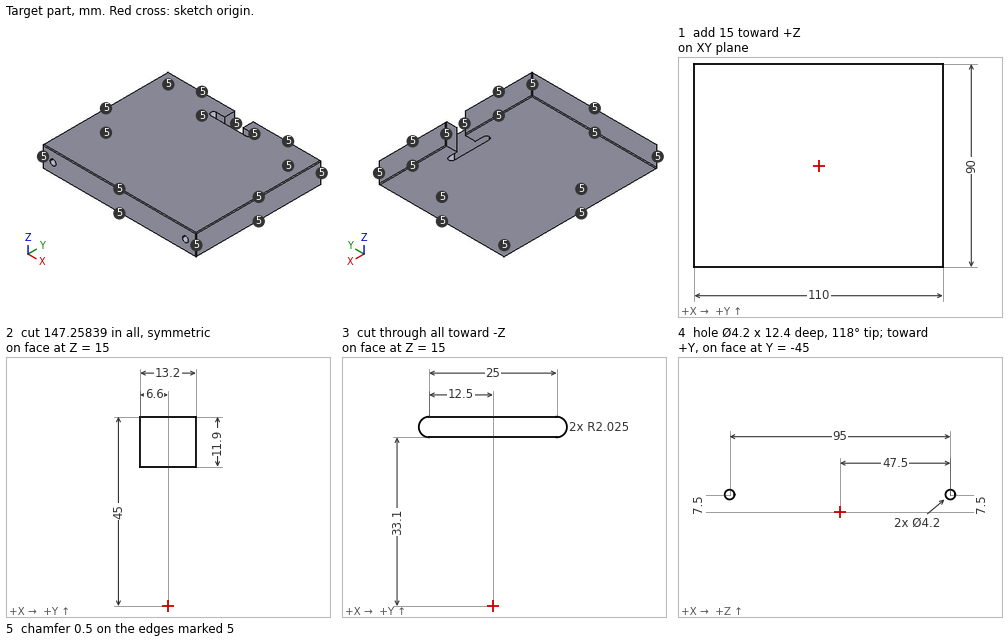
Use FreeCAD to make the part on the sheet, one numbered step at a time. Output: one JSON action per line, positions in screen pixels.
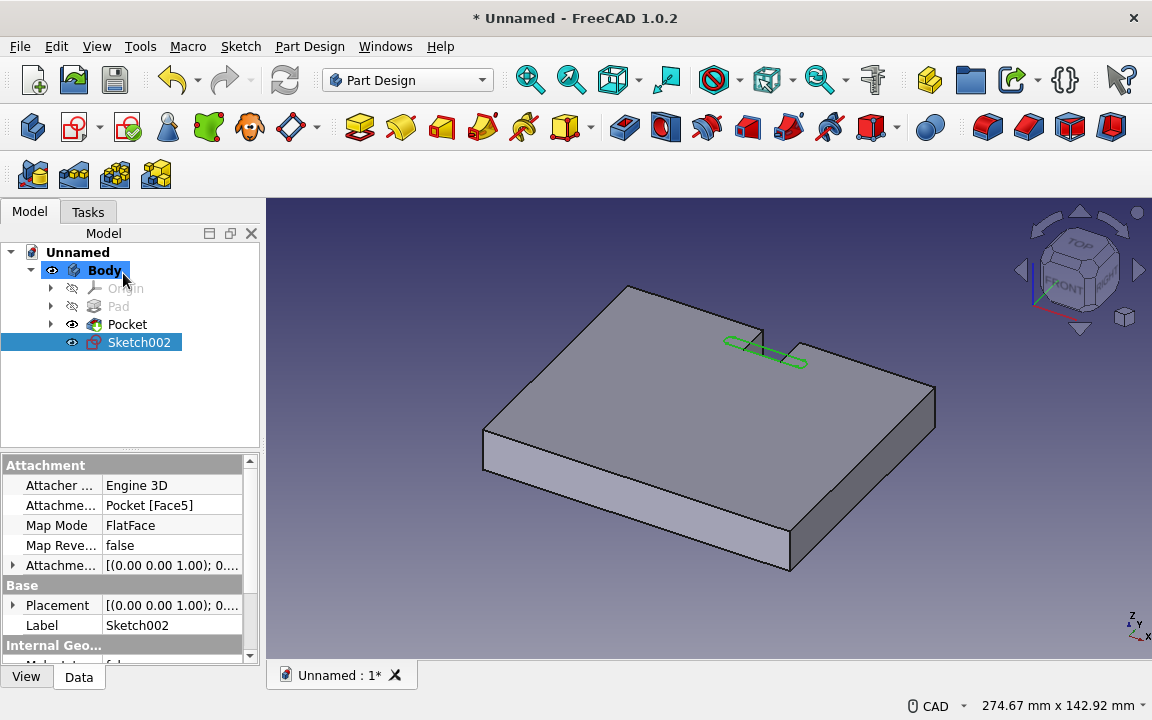
{"action": "left_click", "coordinate": [625, 128]}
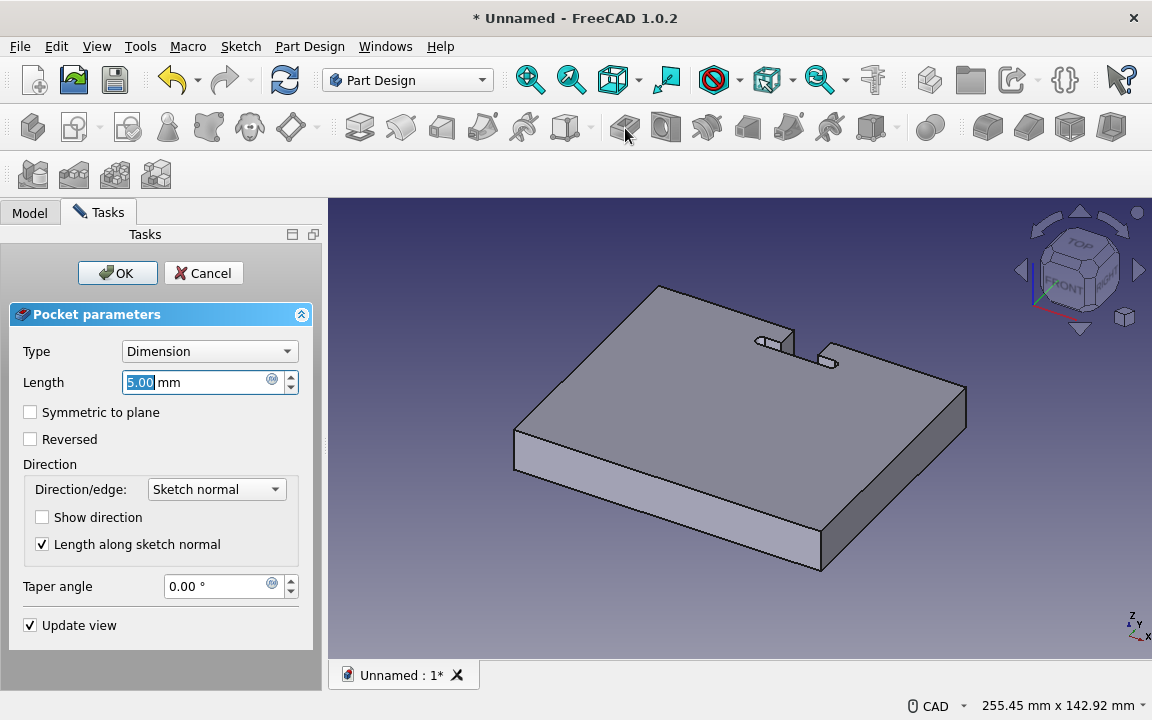
{"action": "left_click", "coordinate": [210, 352]}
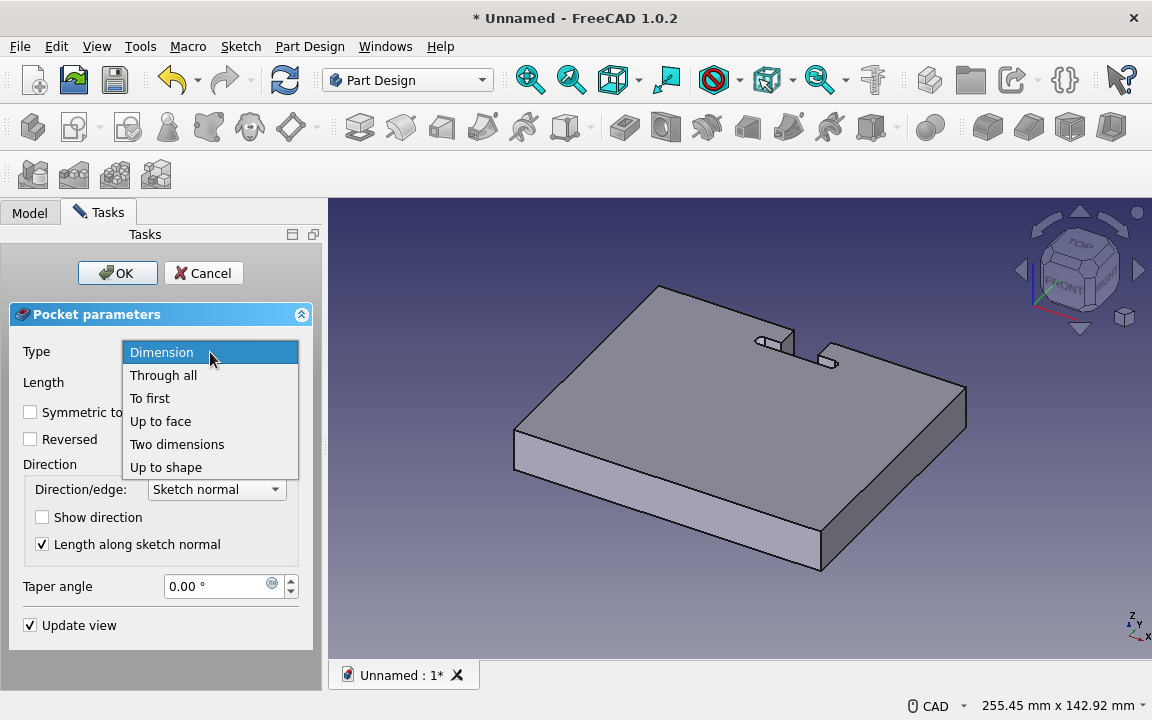
{"action": "left_click", "coordinate": [208, 376]}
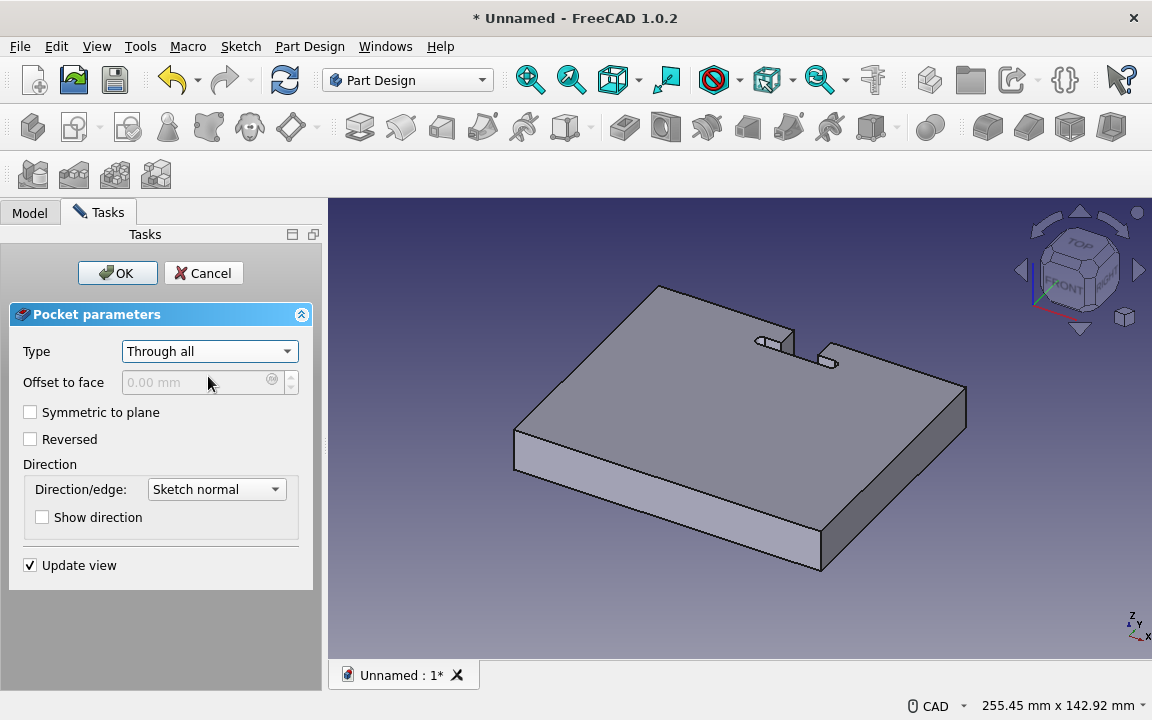
{"action": "left_click", "coordinate": [118, 273]}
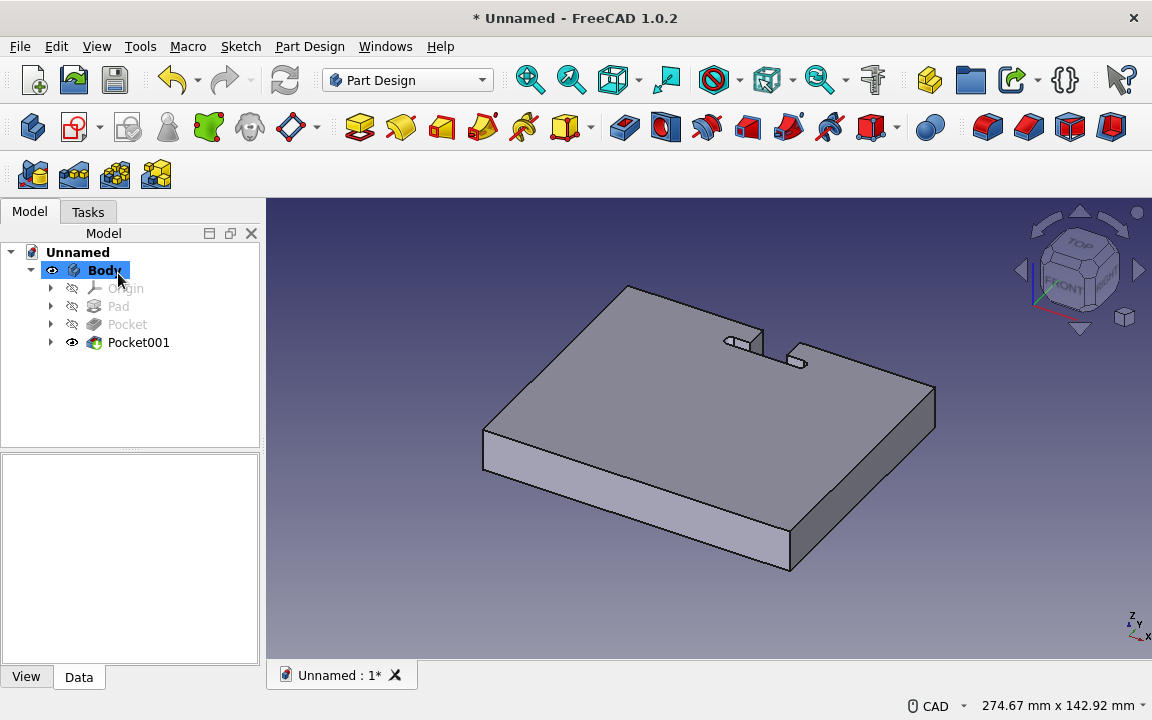
{"action": "left_click", "coordinate": [768, 543]}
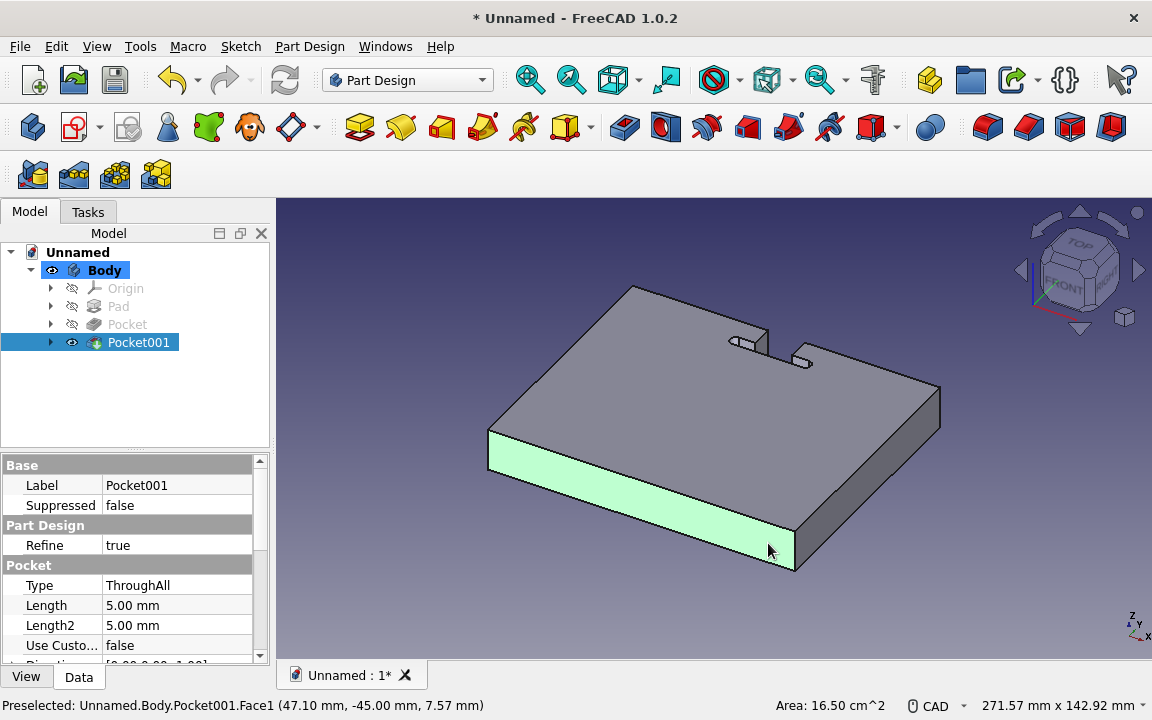
{"action": "left_click", "coordinate": [74, 128]}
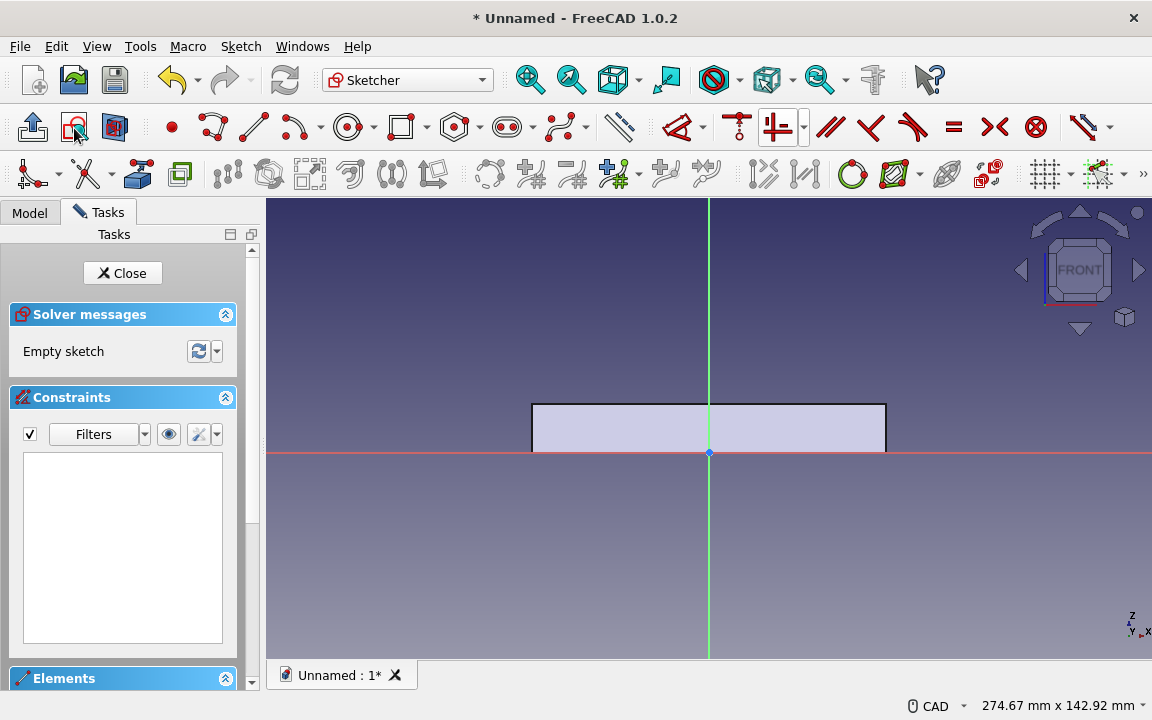
{"action": "scroll", "coordinate": [848, 455], "scroll_direction": "up", "scroll_amount": 2}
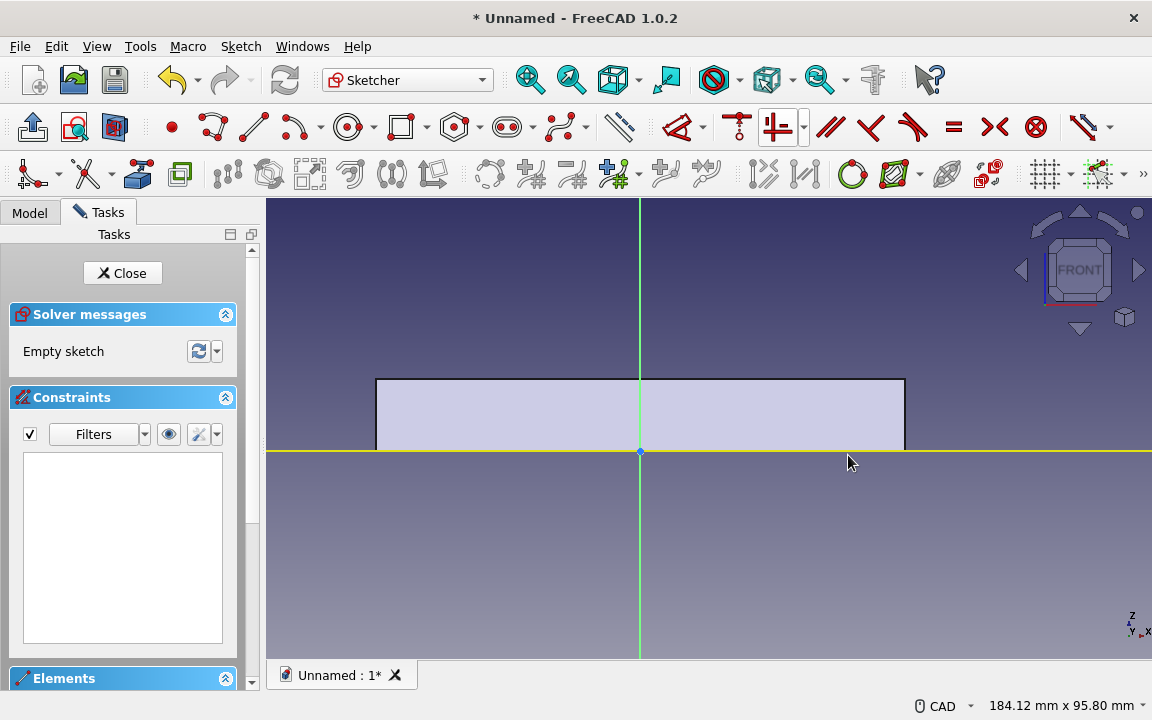
{"action": "left_click", "coordinate": [348, 128]}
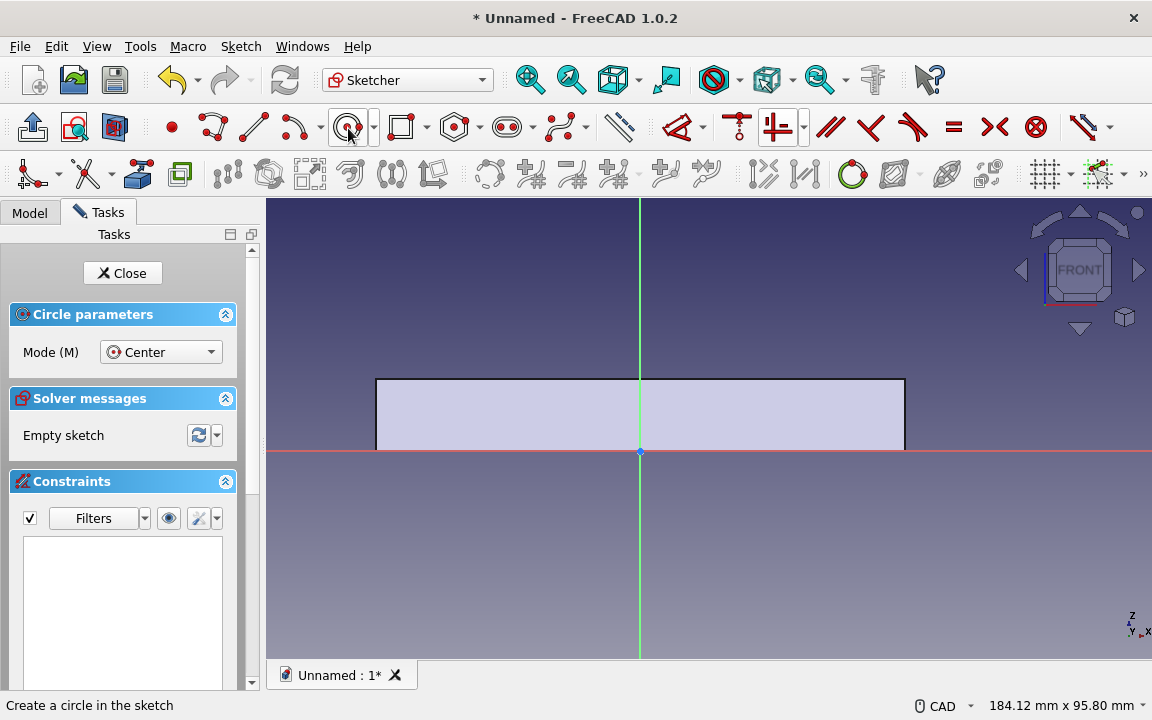
{"action": "scroll", "coordinate": [869, 415], "scroll_direction": "up", "scroll_amount": 5}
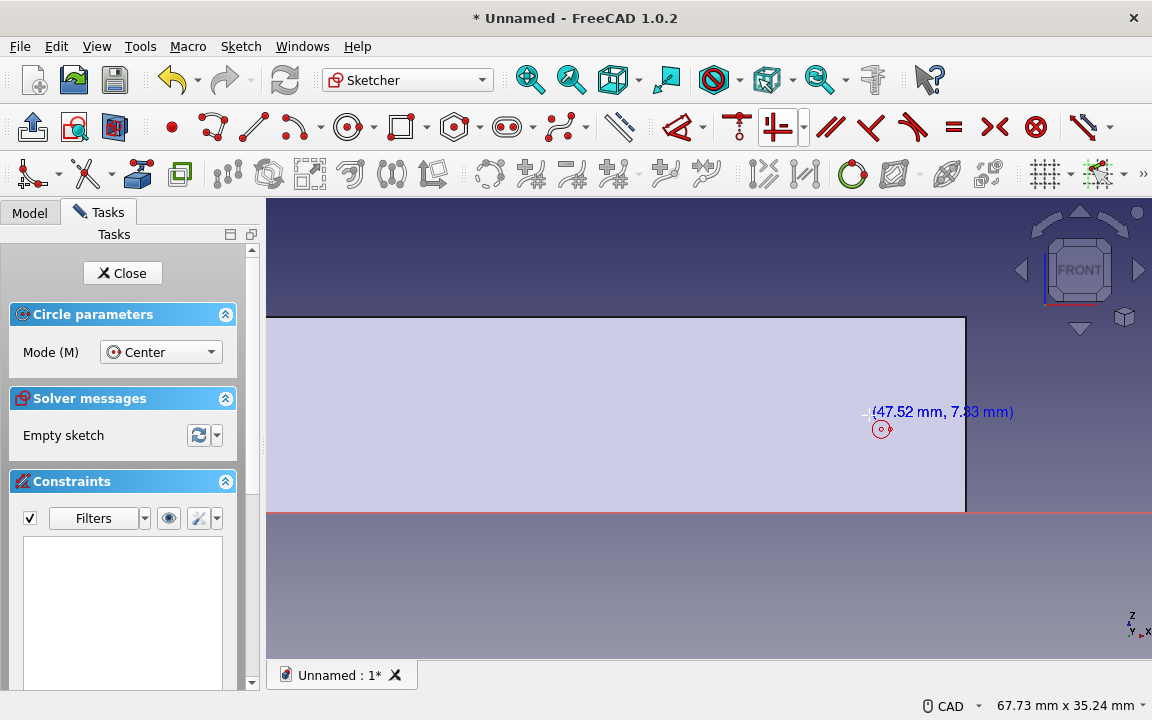
{"action": "left_click", "coordinate": [868, 415]}
{"action": "mouse_move", "coordinate": [887, 395]}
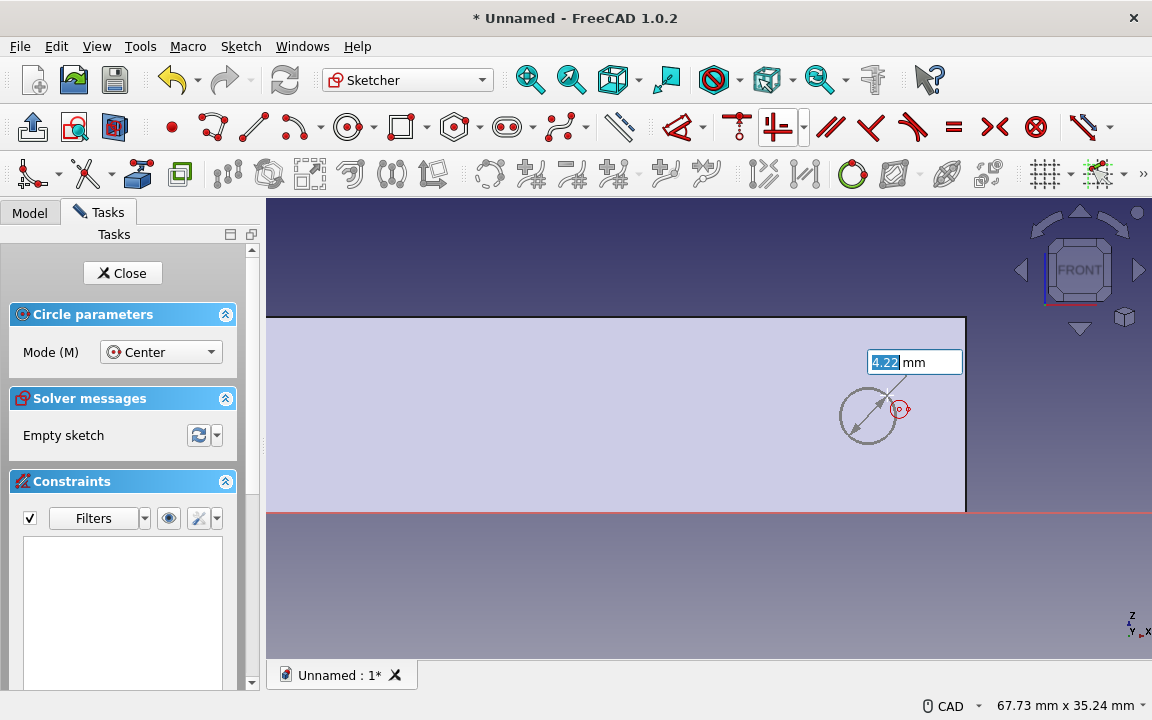
{"action": "type", "text": "4.2"}
{"action": "key", "text": "Return"}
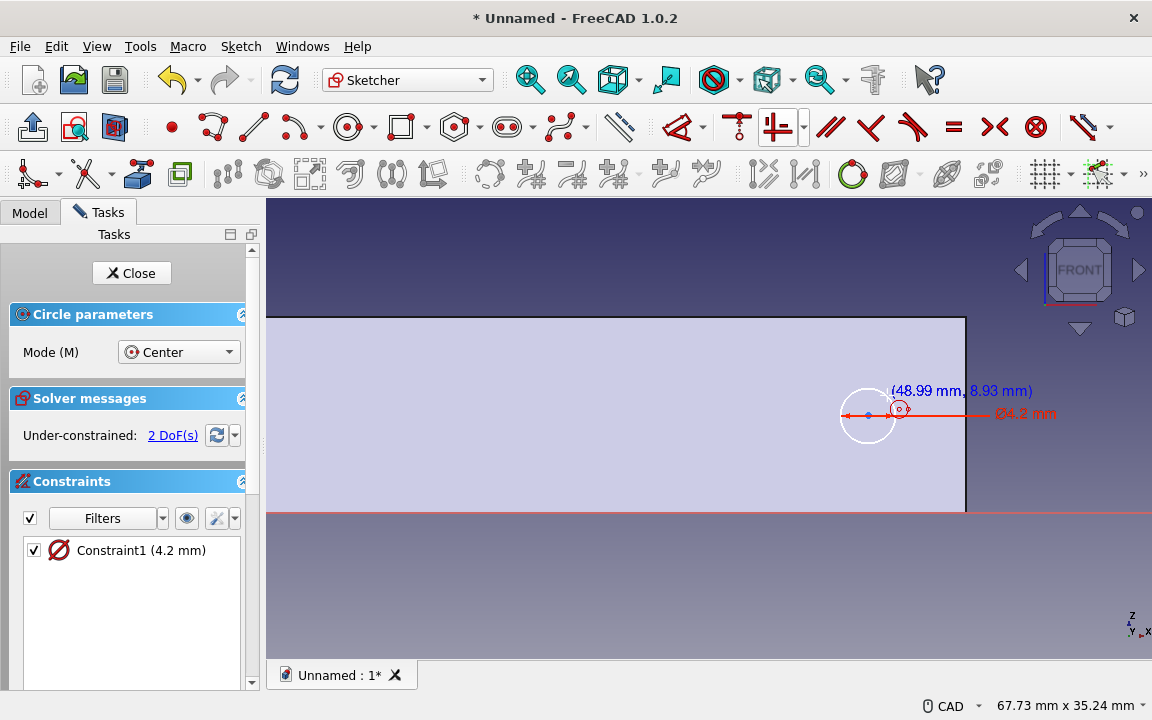
{"action": "scroll", "coordinate": [870, 416], "scroll_direction": "down", "scroll_amount": 5}